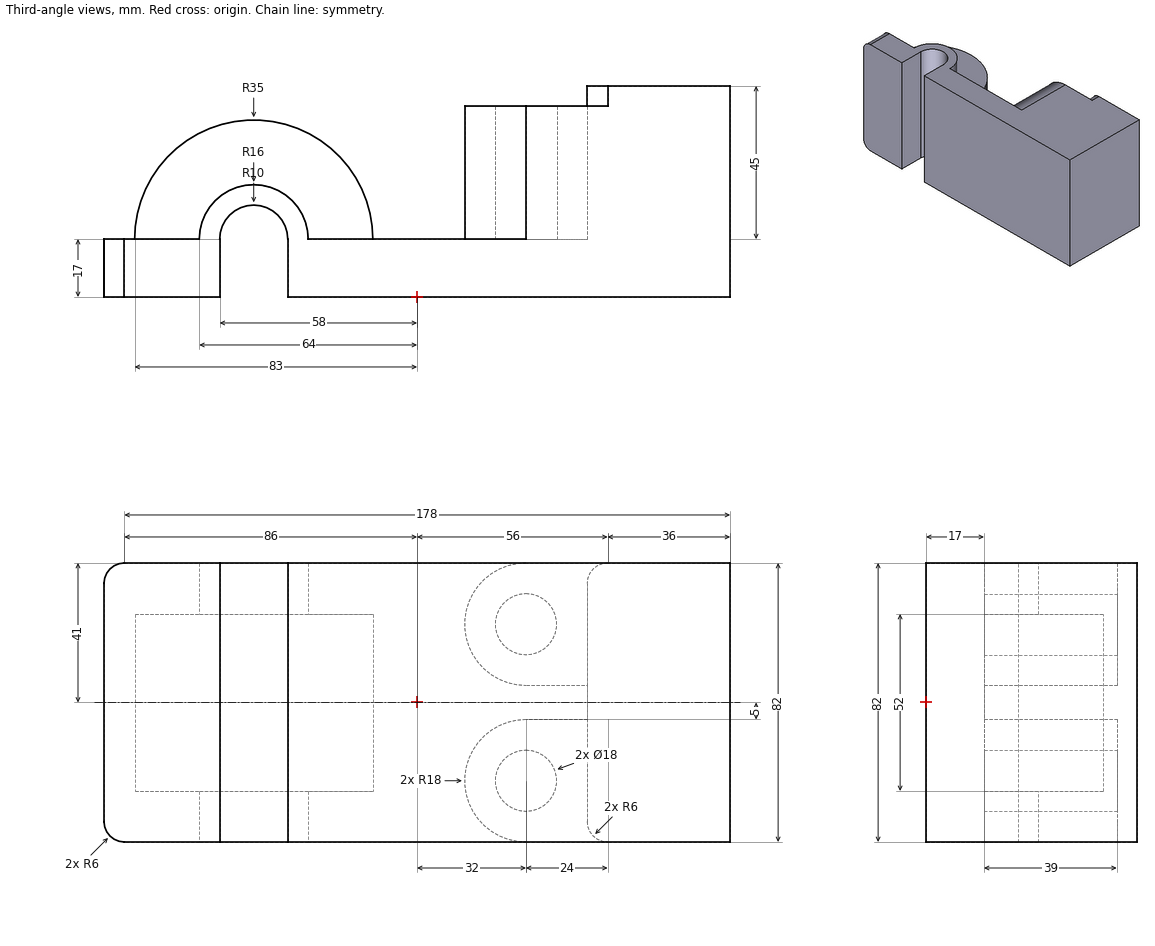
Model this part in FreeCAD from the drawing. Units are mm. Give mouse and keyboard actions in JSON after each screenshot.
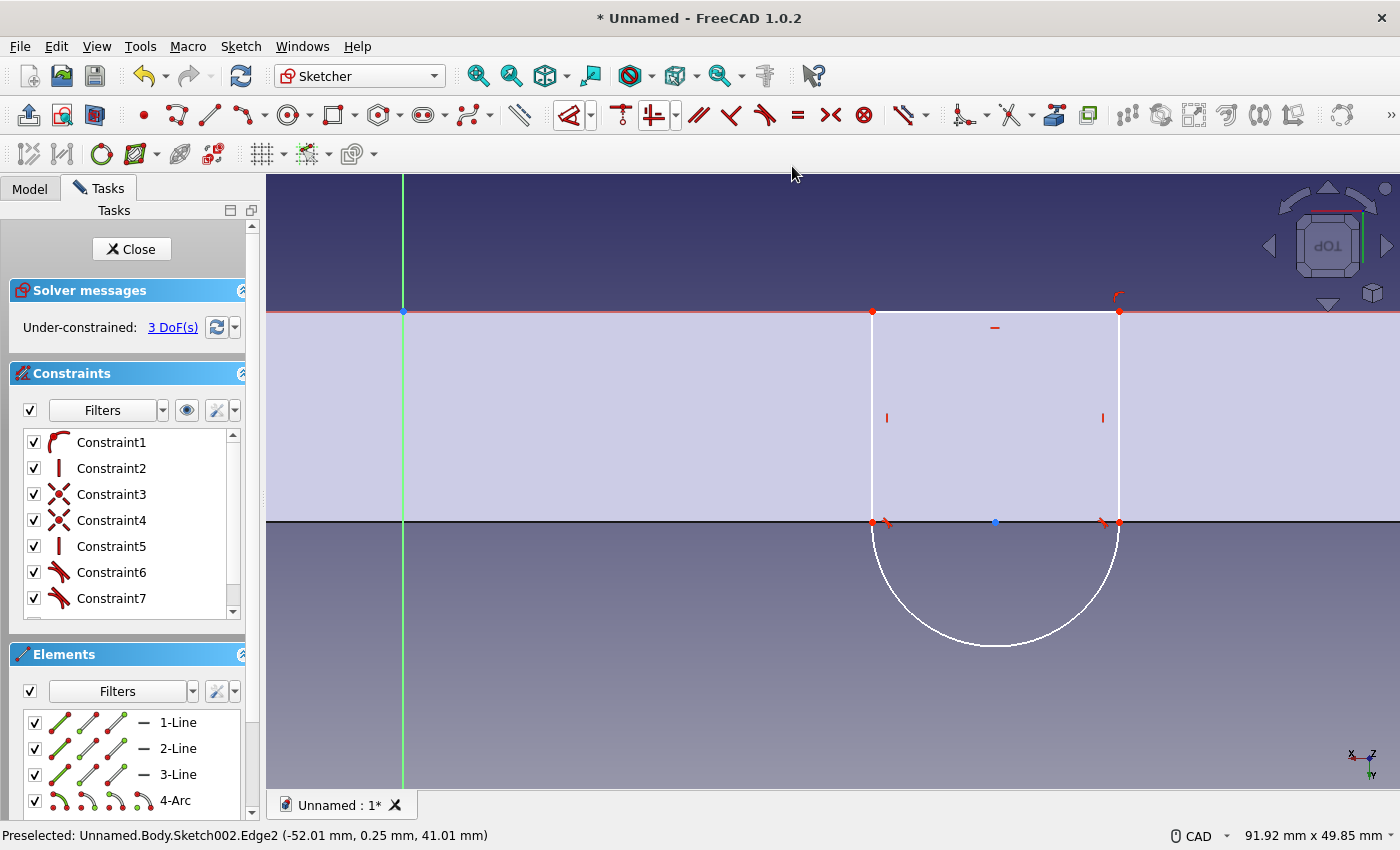
{"action": "left_click", "coordinate": [923, 623]}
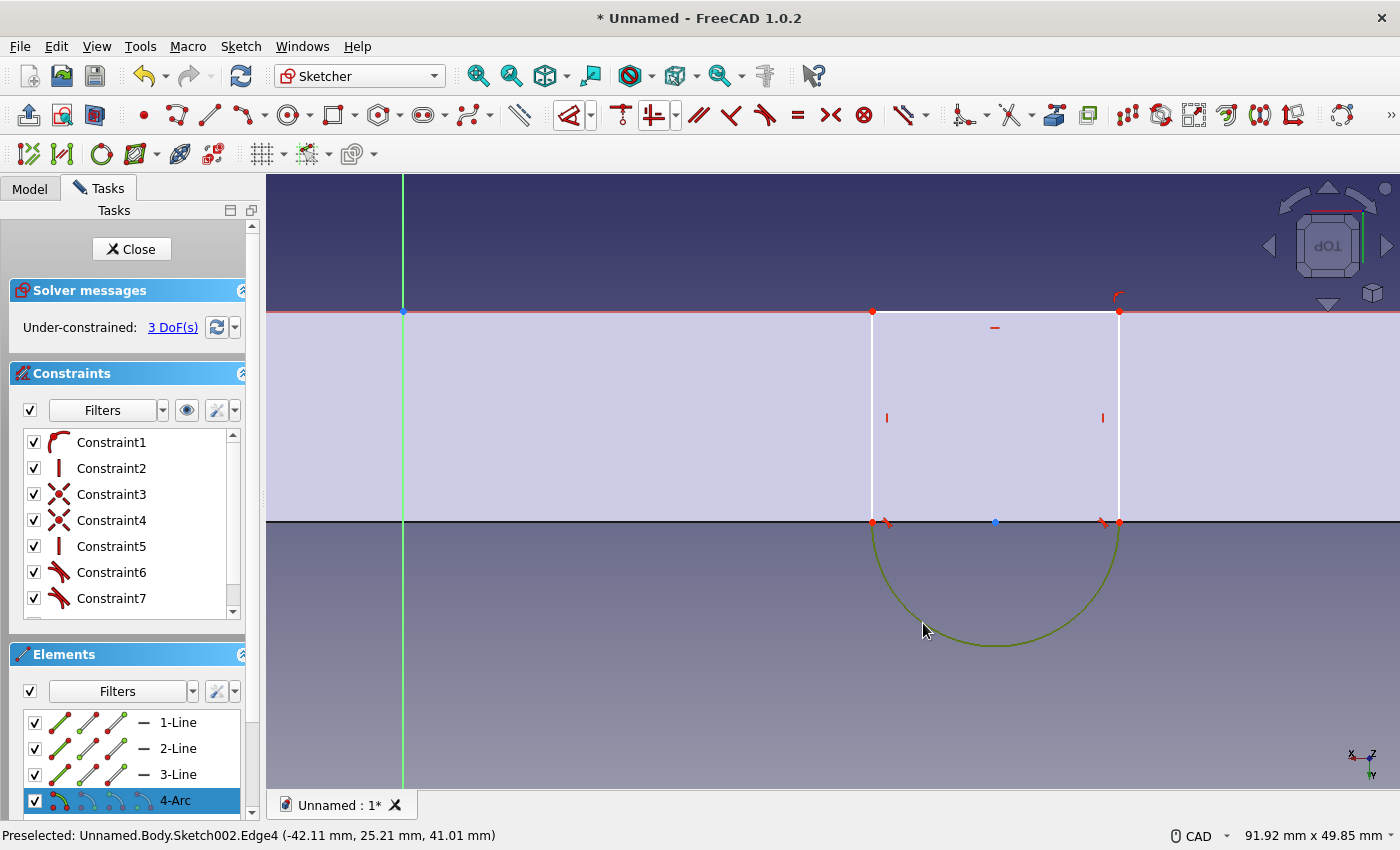
{"action": "left_click", "coordinate": [590, 116]}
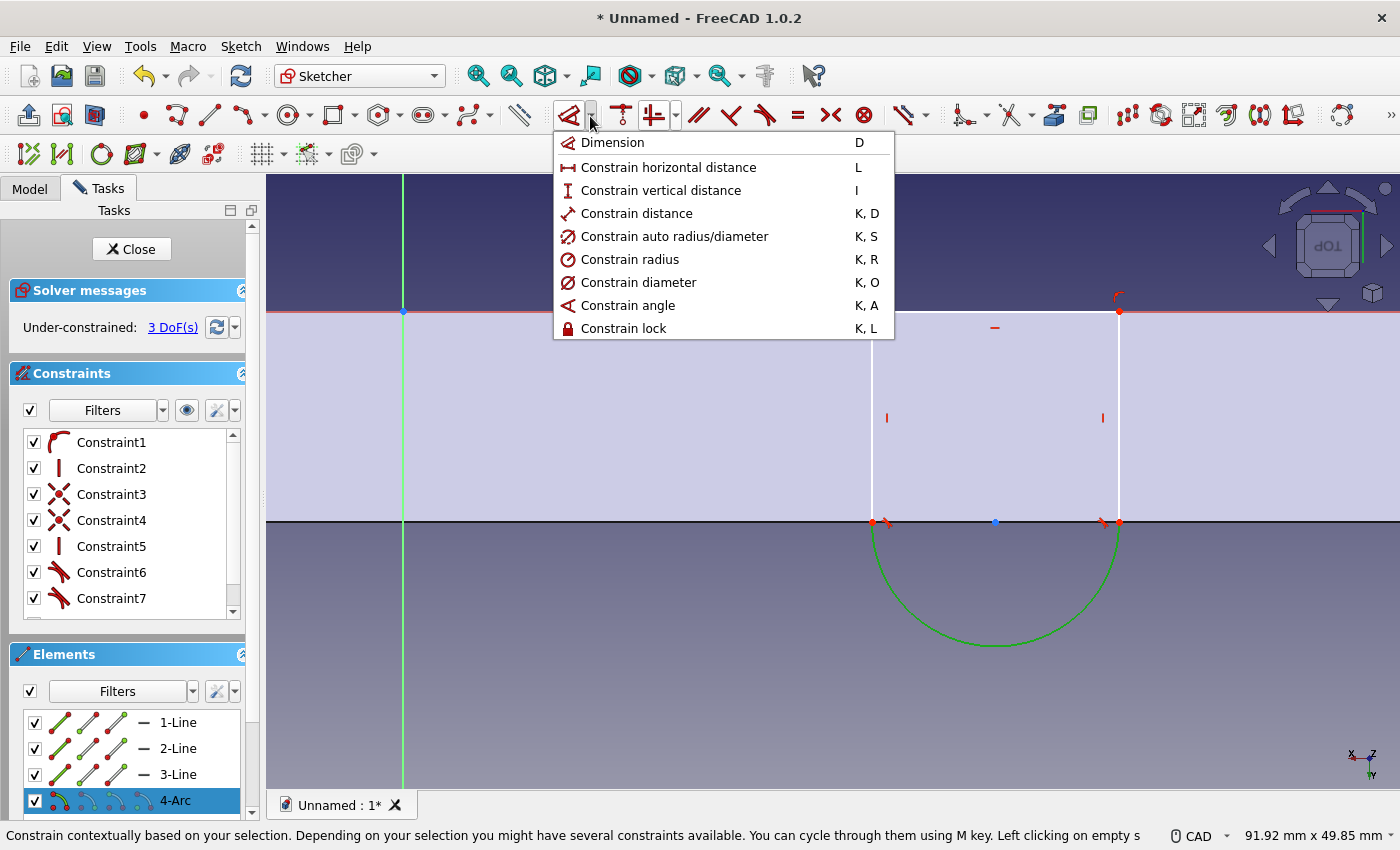
{"action": "left_click", "coordinate": [724, 260]}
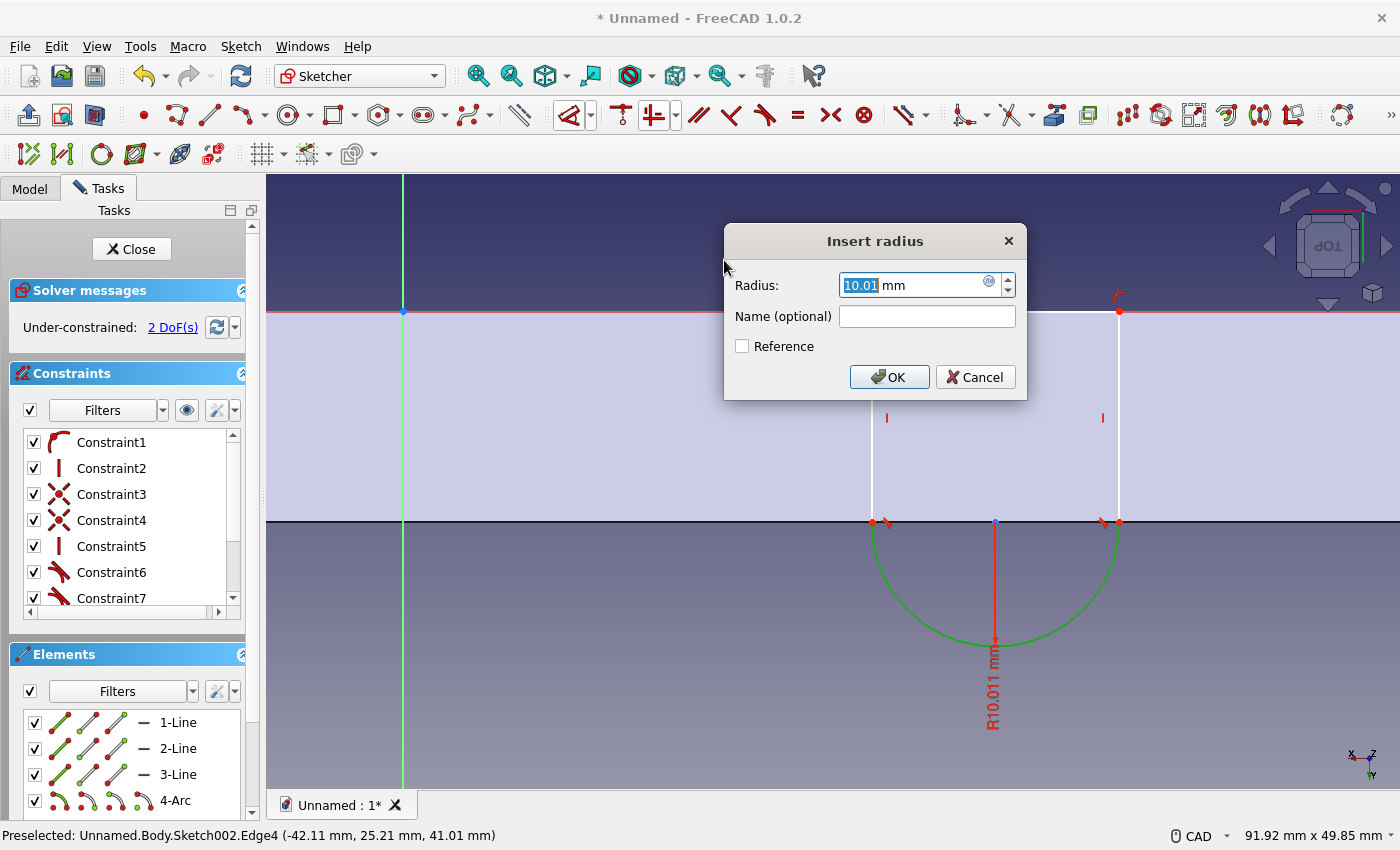
{"action": "type", "text": "10"}
{"action": "key", "text": "Return"}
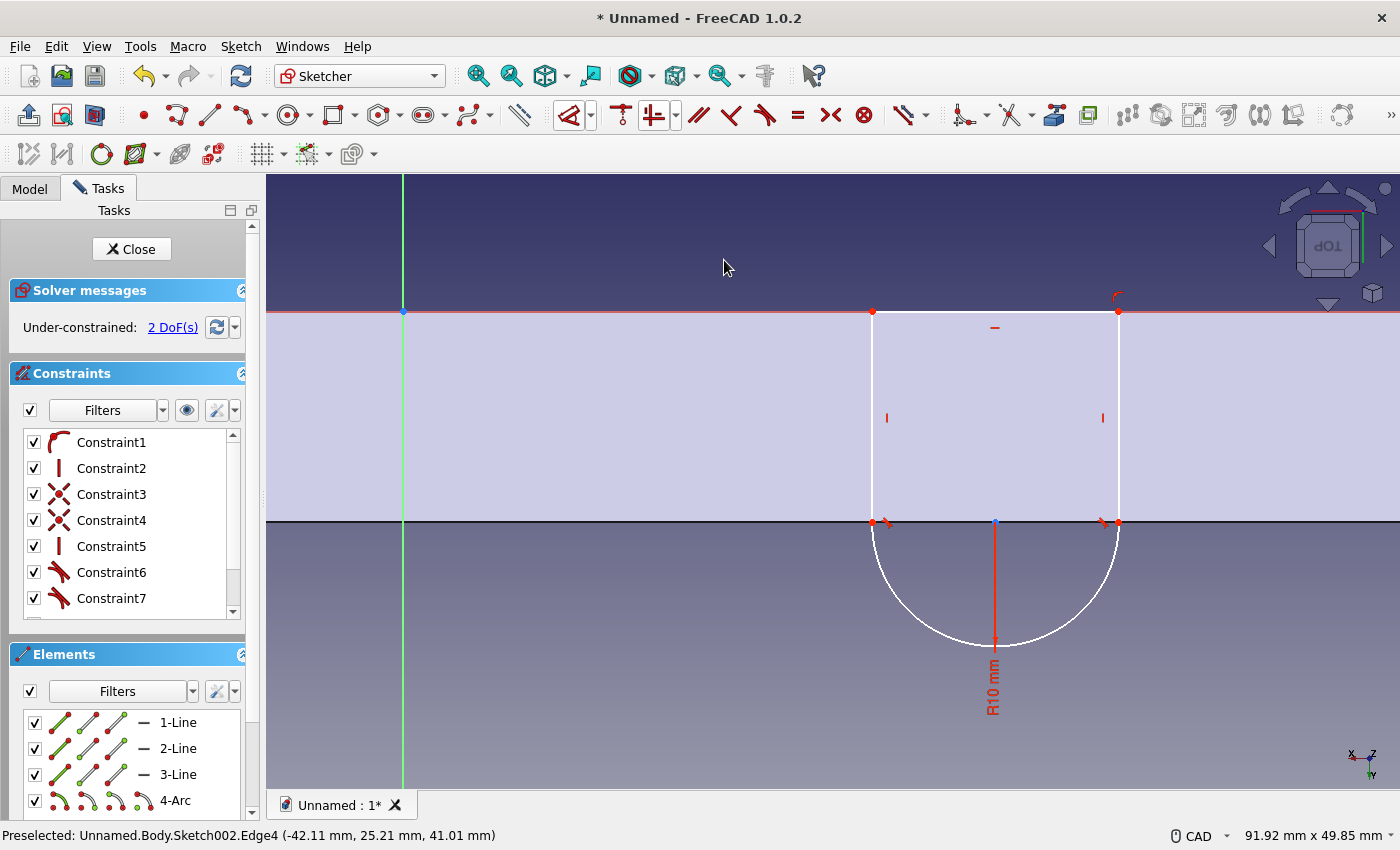
{"action": "left_click", "coordinate": [1119, 460]}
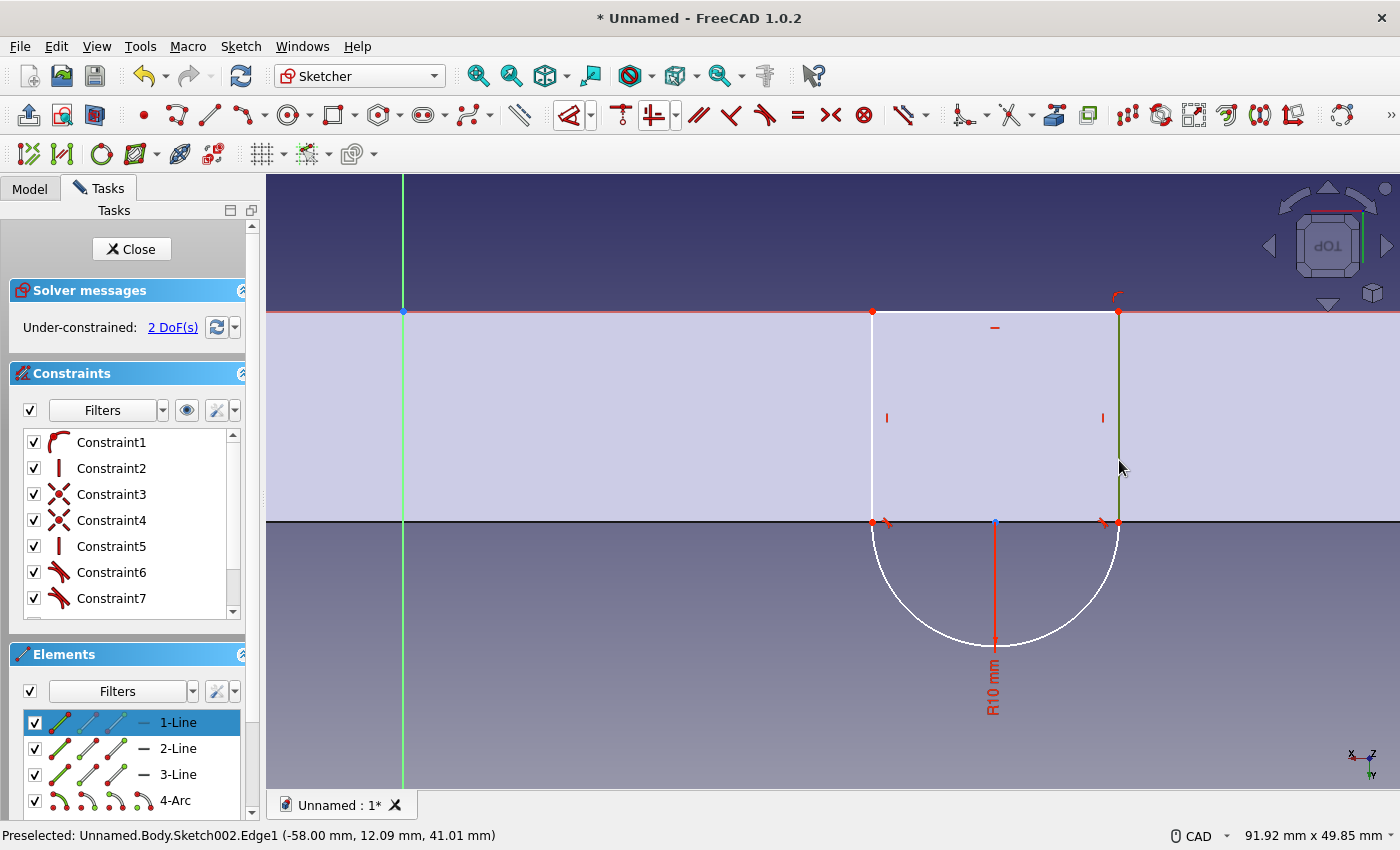
{"action": "left_click", "coordinate": [590, 116]}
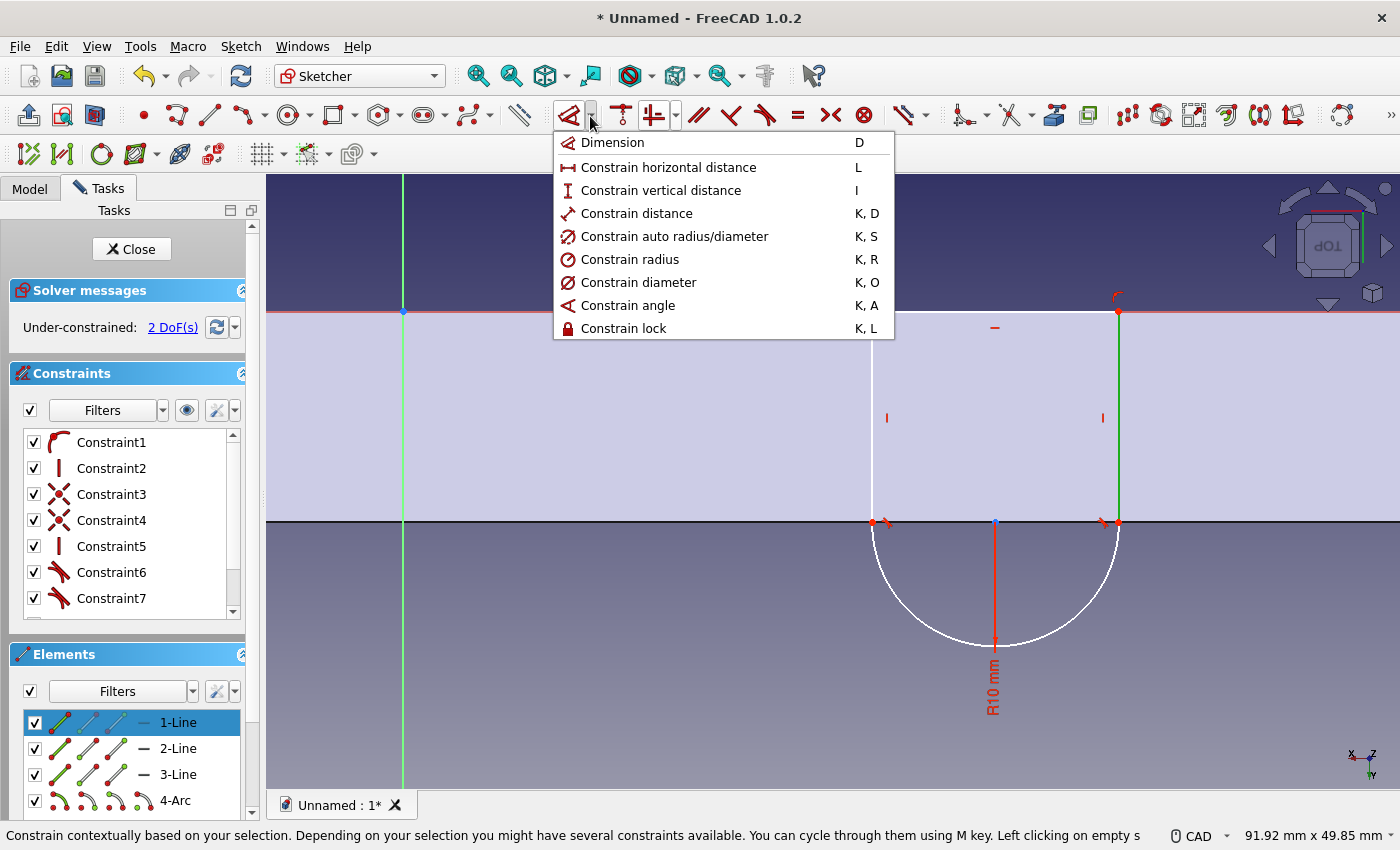
{"action": "left_click", "coordinate": [724, 190]}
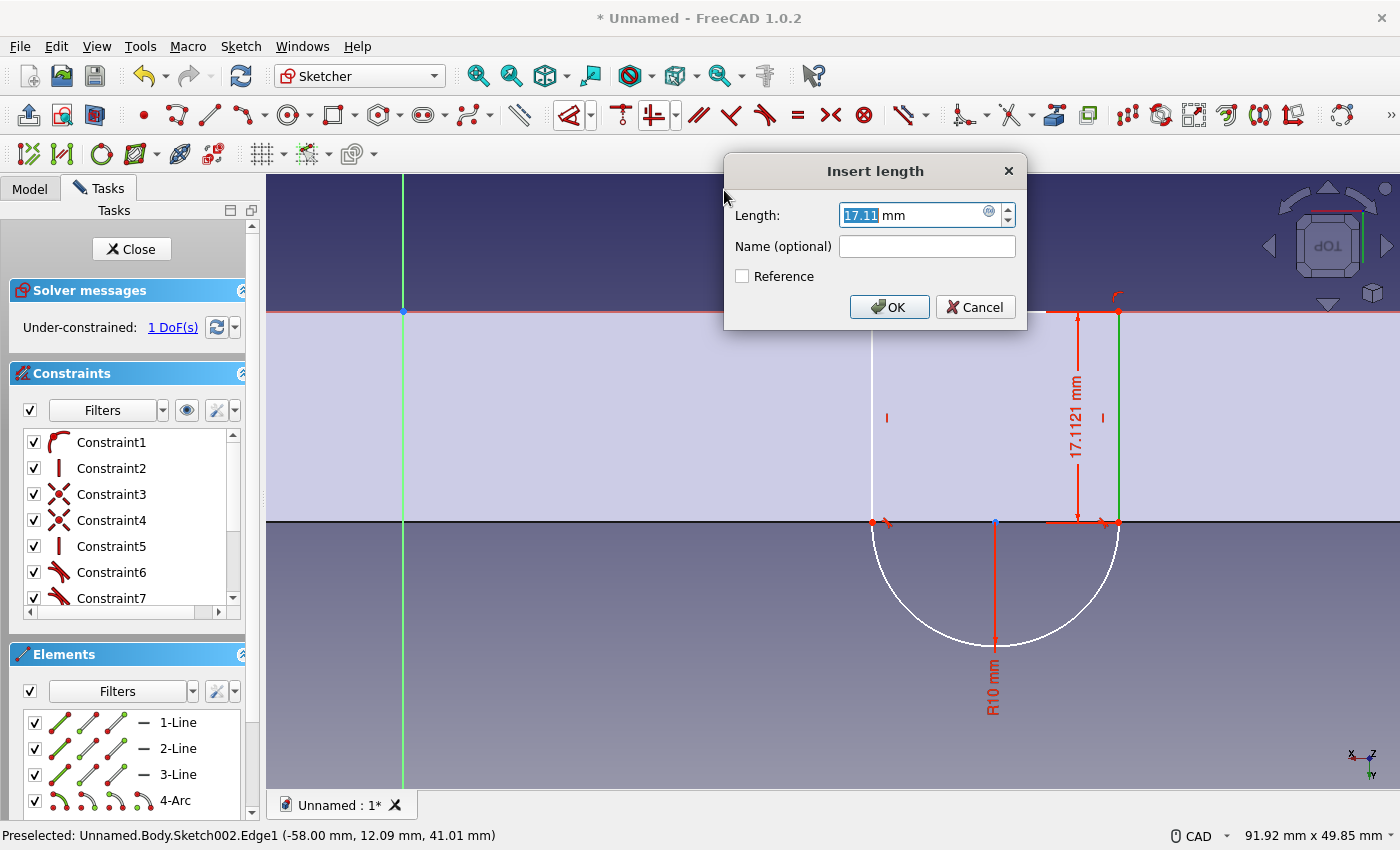
{"action": "type", "text": "17"}
{"action": "key", "text": "Return"}